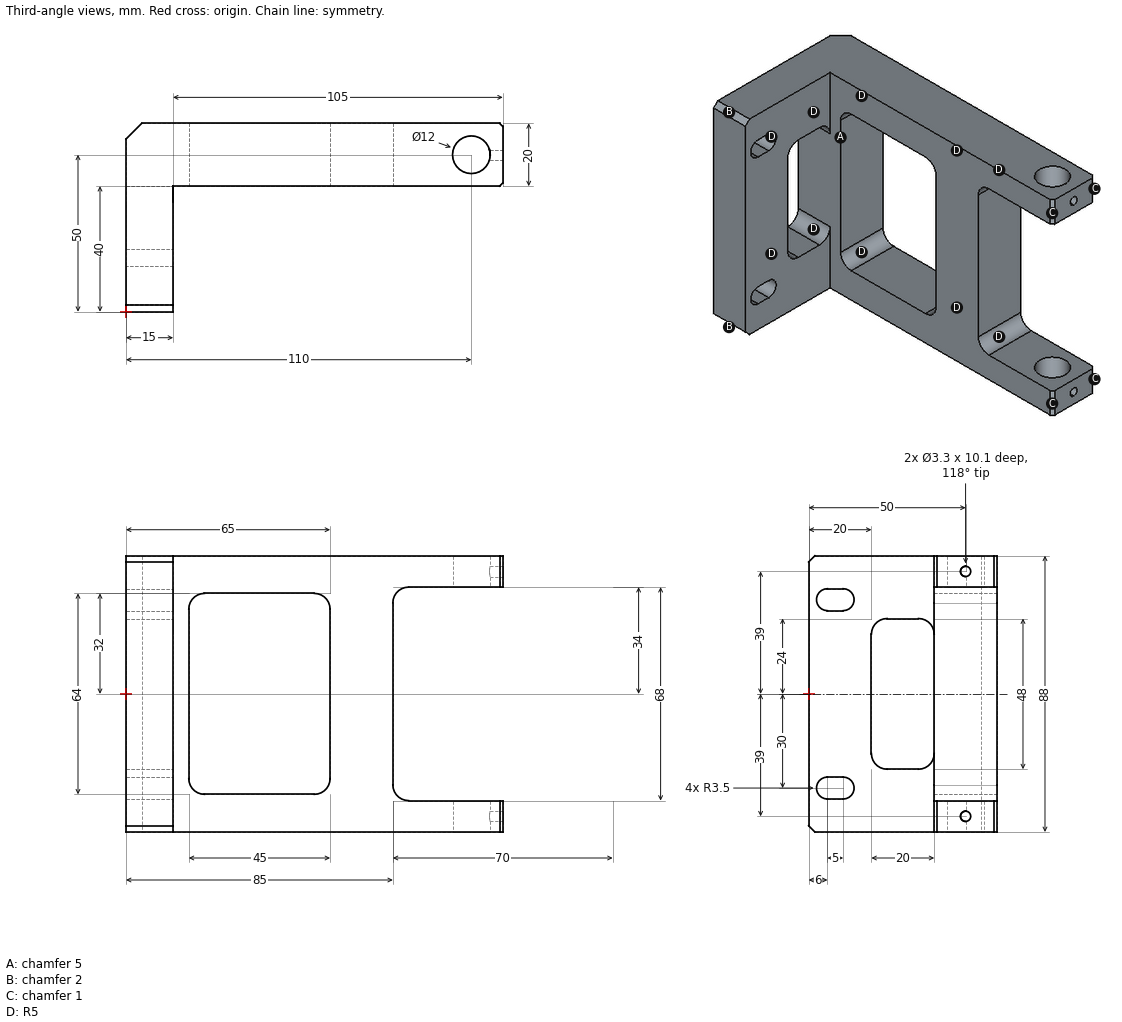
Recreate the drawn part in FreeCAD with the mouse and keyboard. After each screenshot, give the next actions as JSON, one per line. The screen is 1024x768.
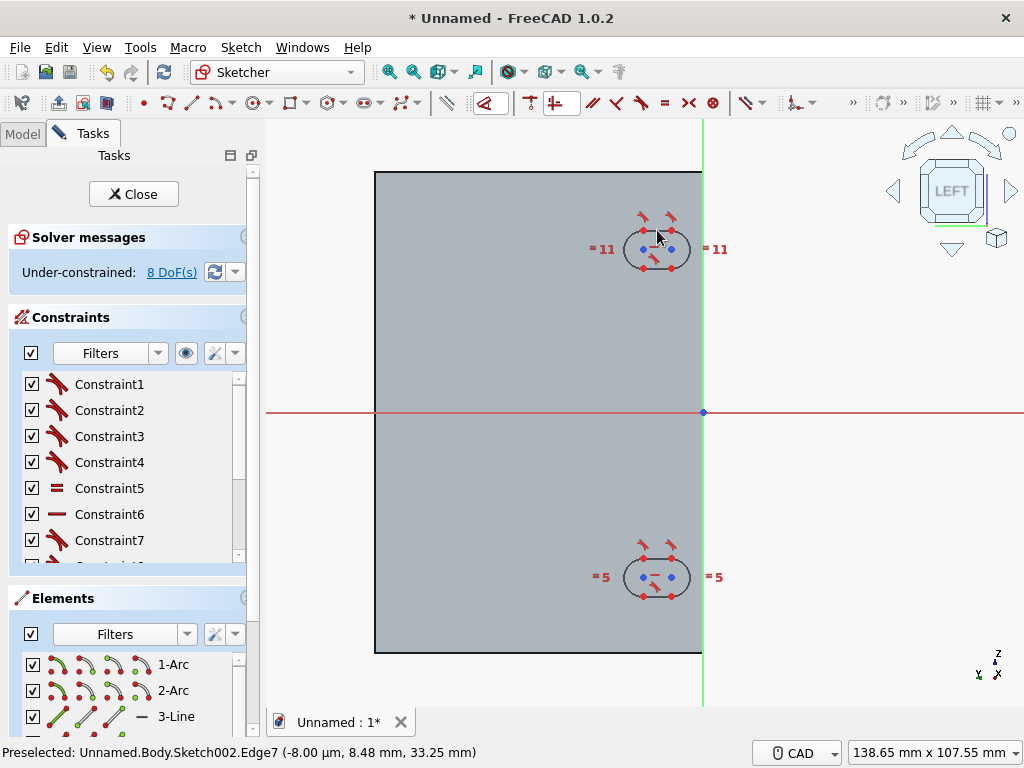
{"action": "left_click", "coordinate": [628, 567]}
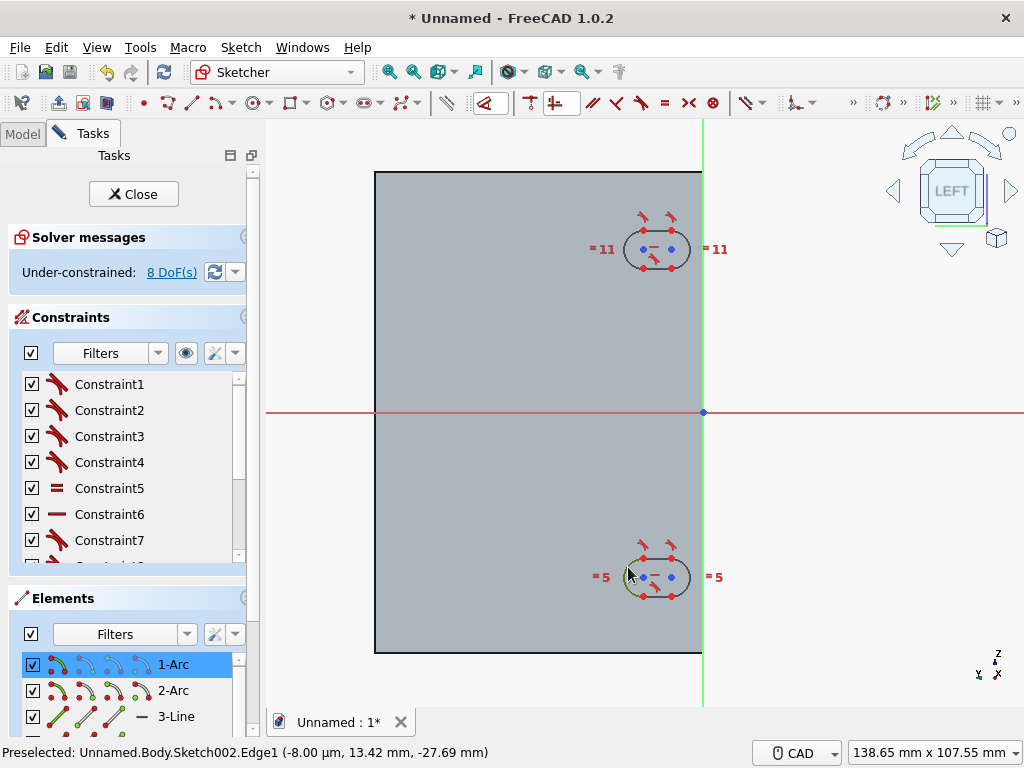
{"action": "left_click", "coordinate": [628, 239]}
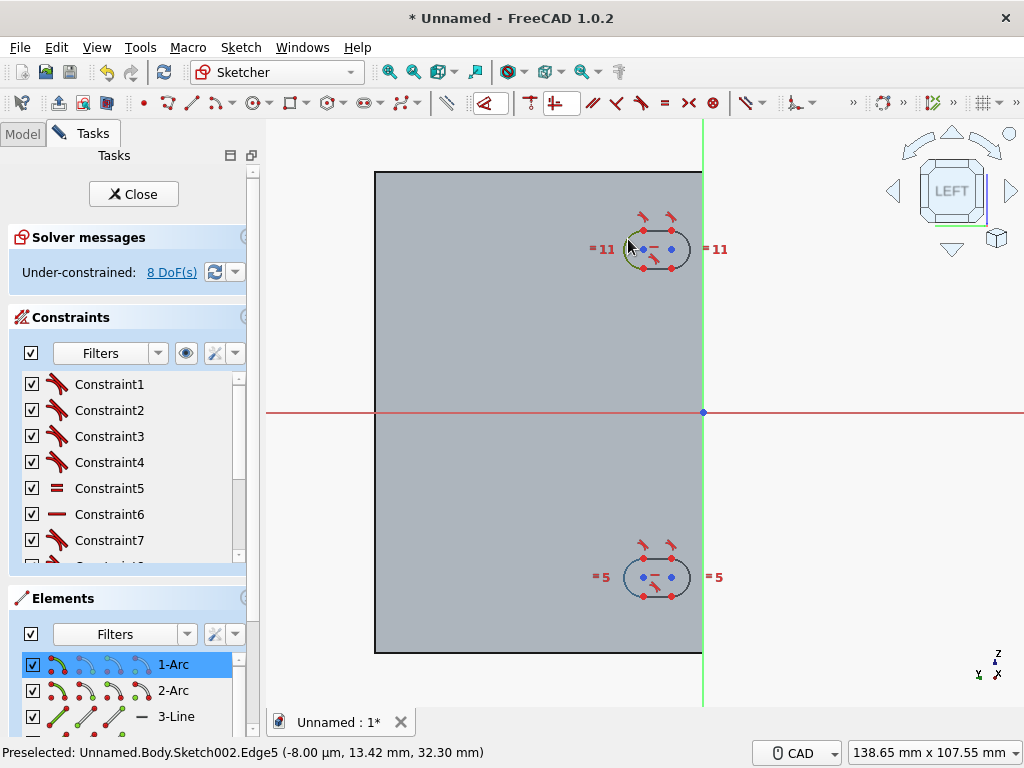
{"action": "key", "text": "e"}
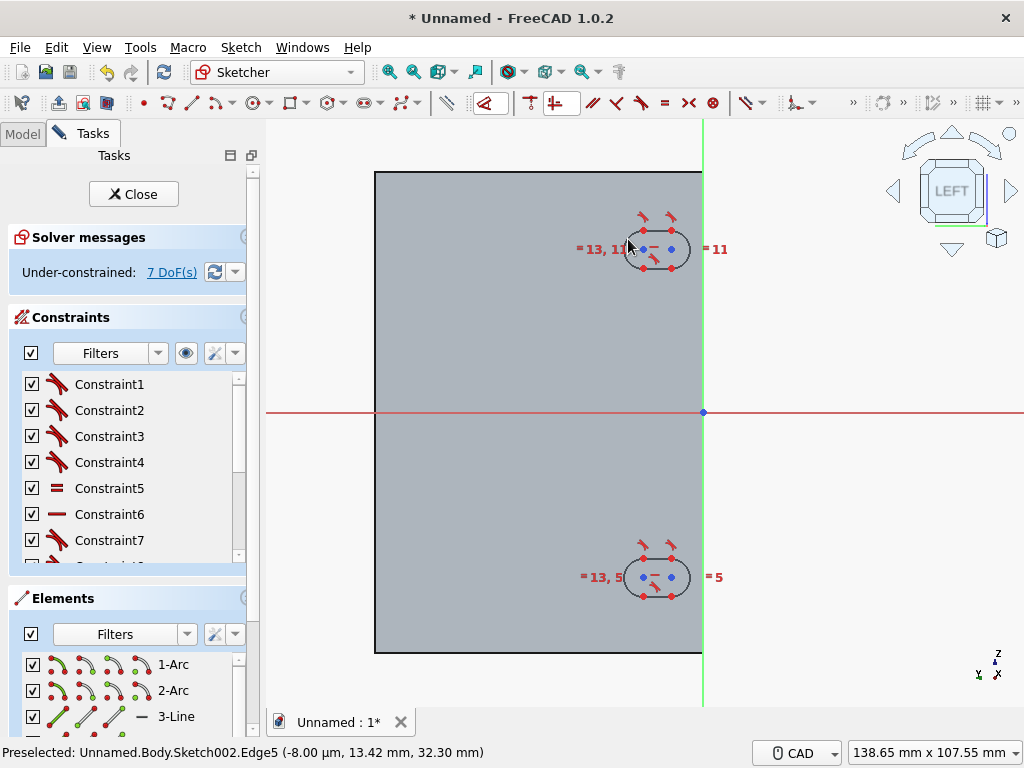
{"action": "left_click", "coordinate": [643, 578]}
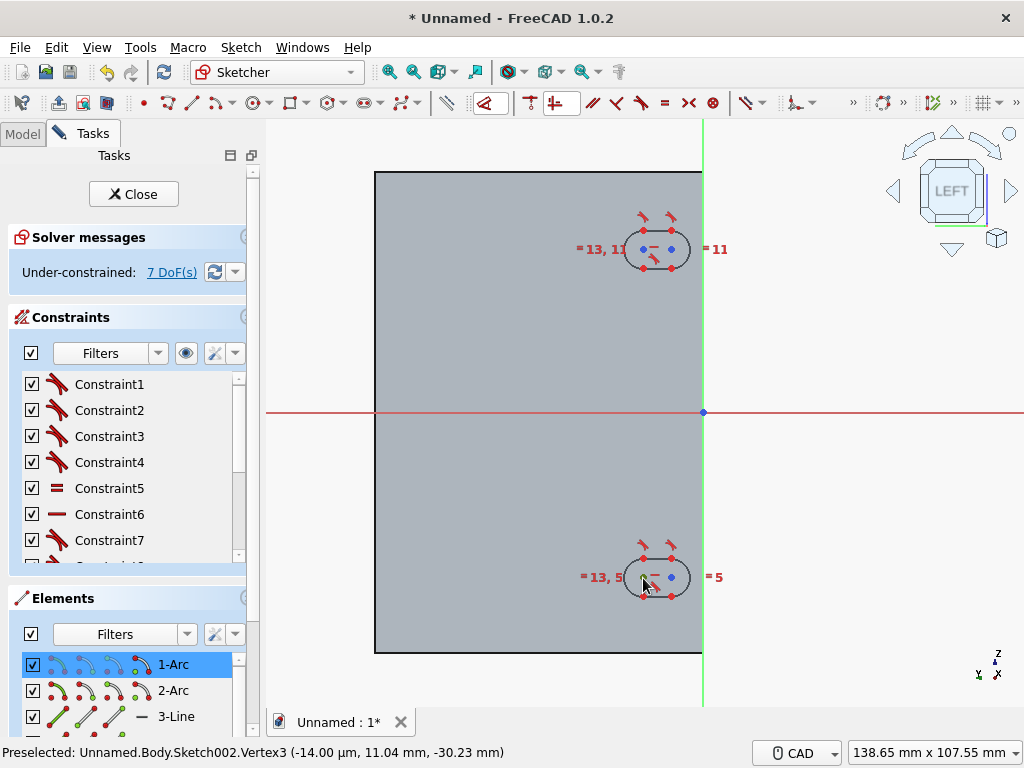
{"action": "left_click", "coordinate": [643, 250]}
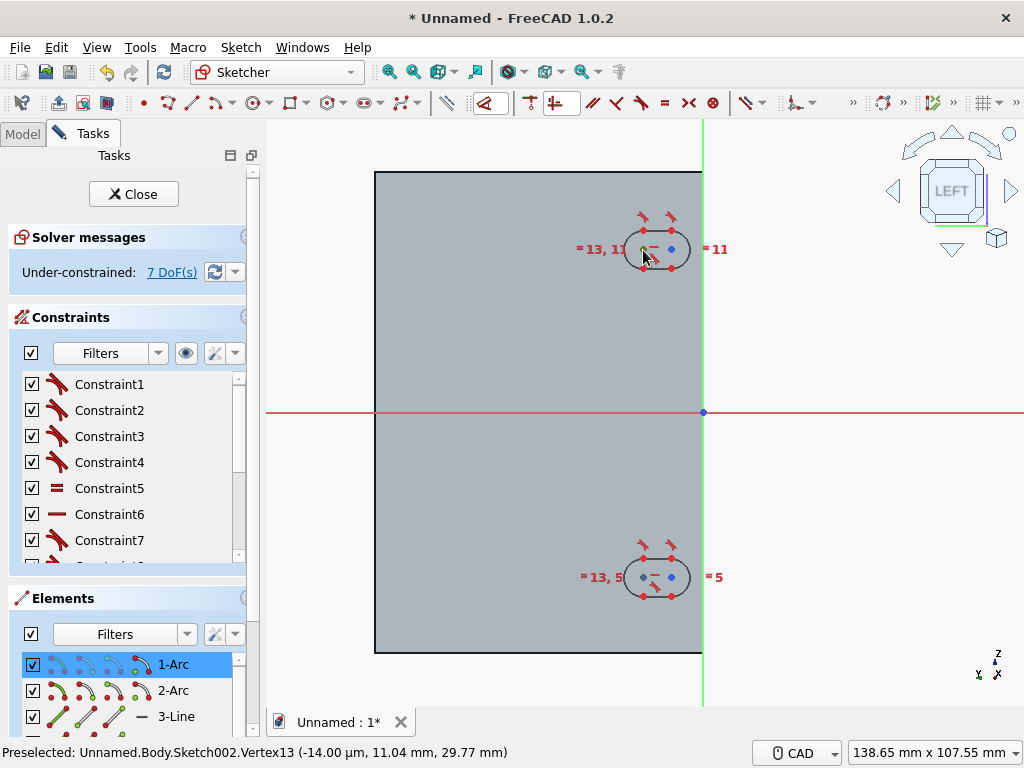
{"action": "left_click", "coordinate": [334, 413]}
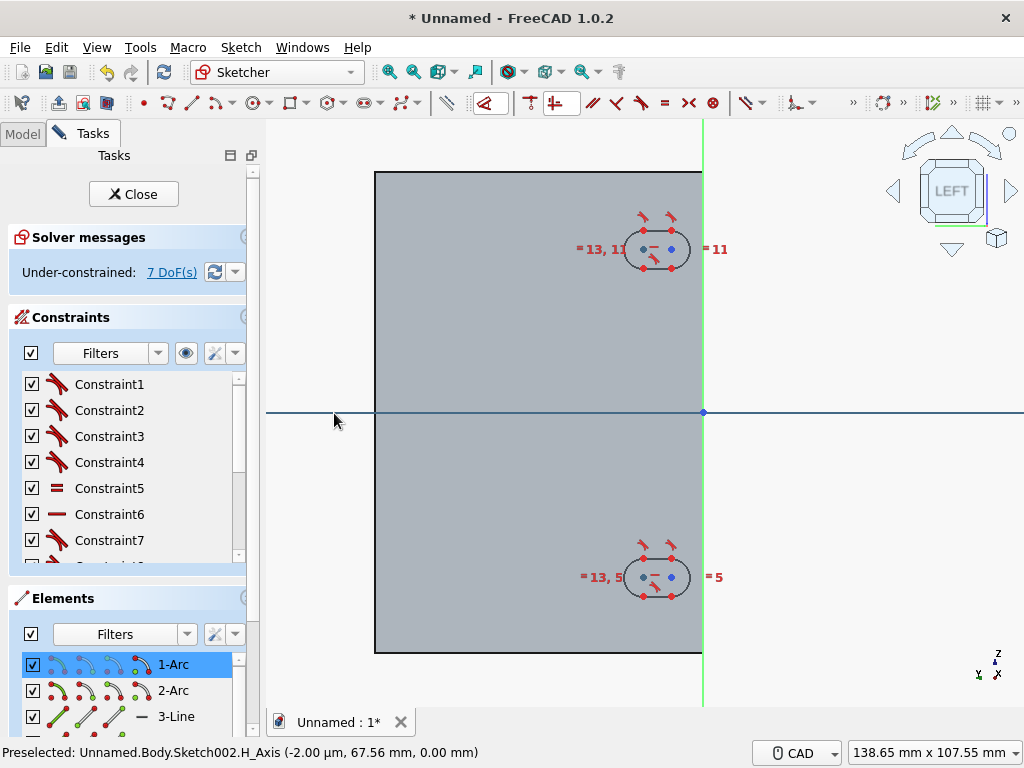
{"action": "key", "text": "s"}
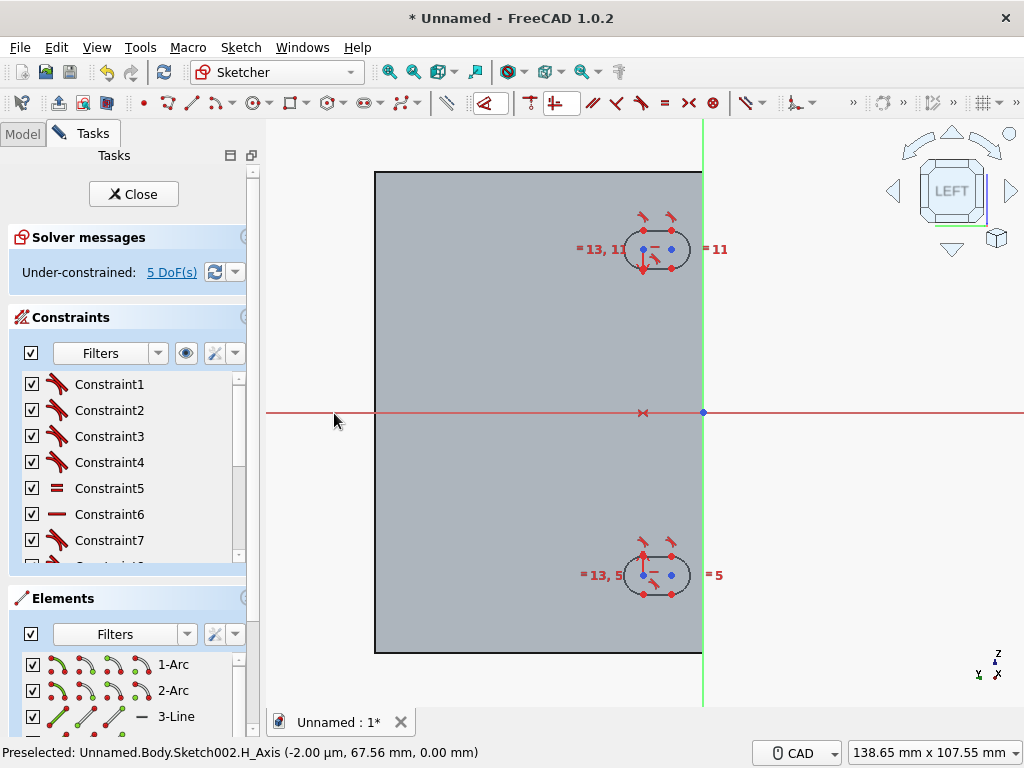
{"action": "scroll", "coordinate": [628, 564], "scroll_direction": "up", "scroll_amount": 4}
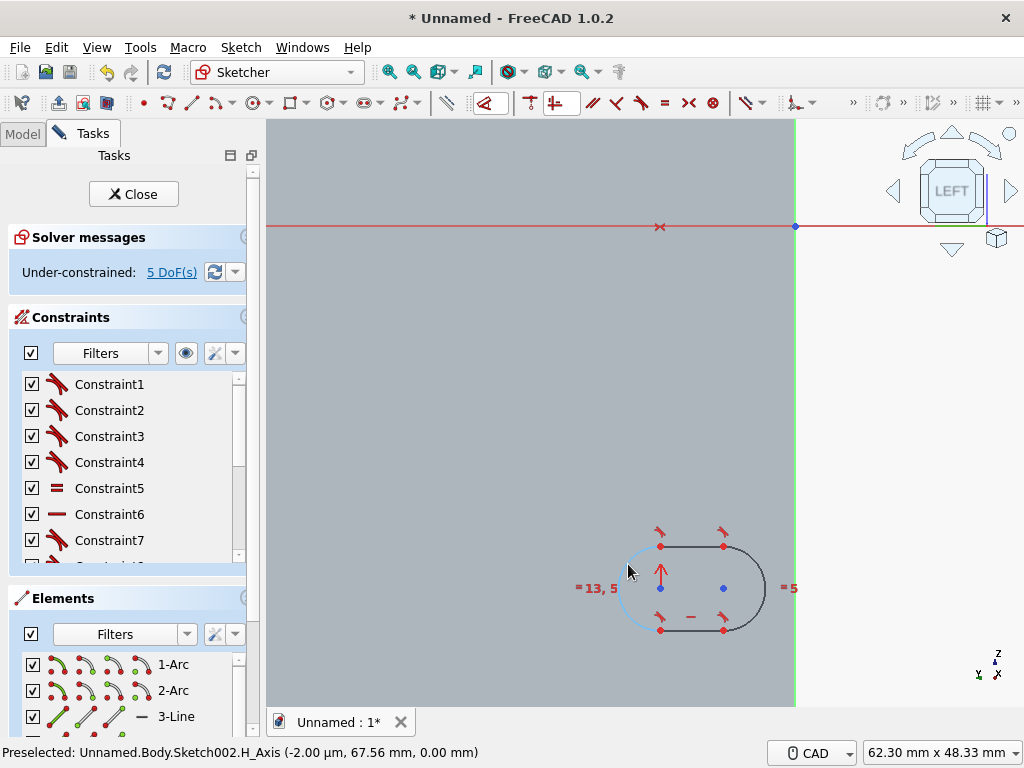
{"action": "left_click", "coordinate": [627, 564]}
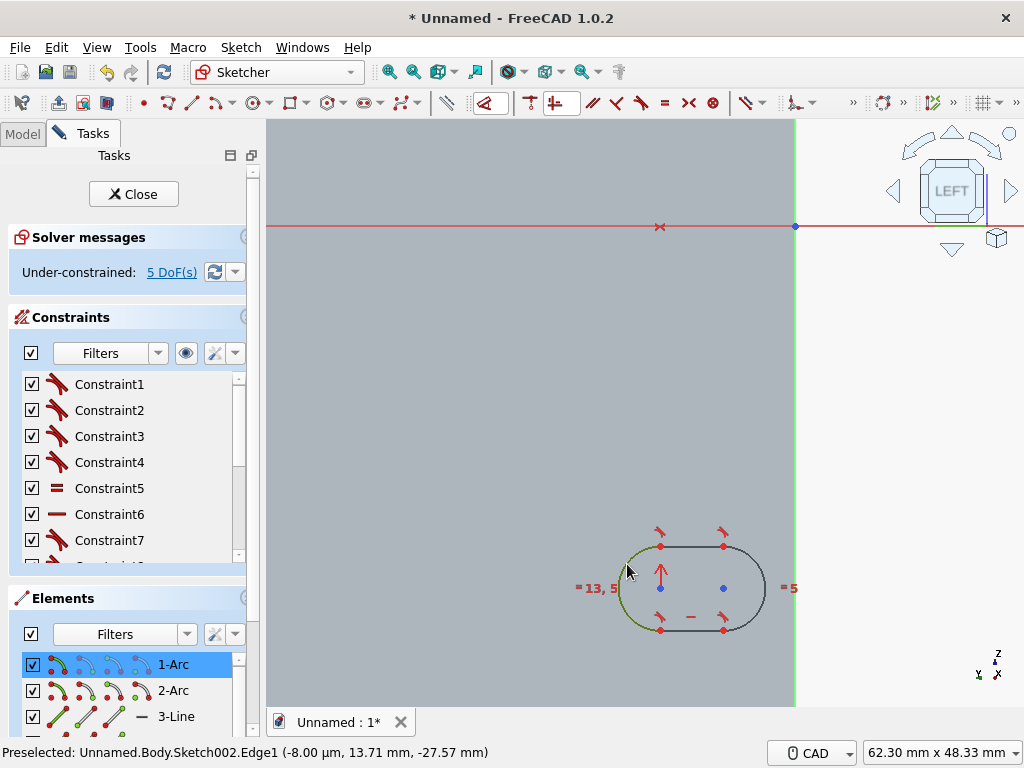
{"action": "key", "text": "k r"}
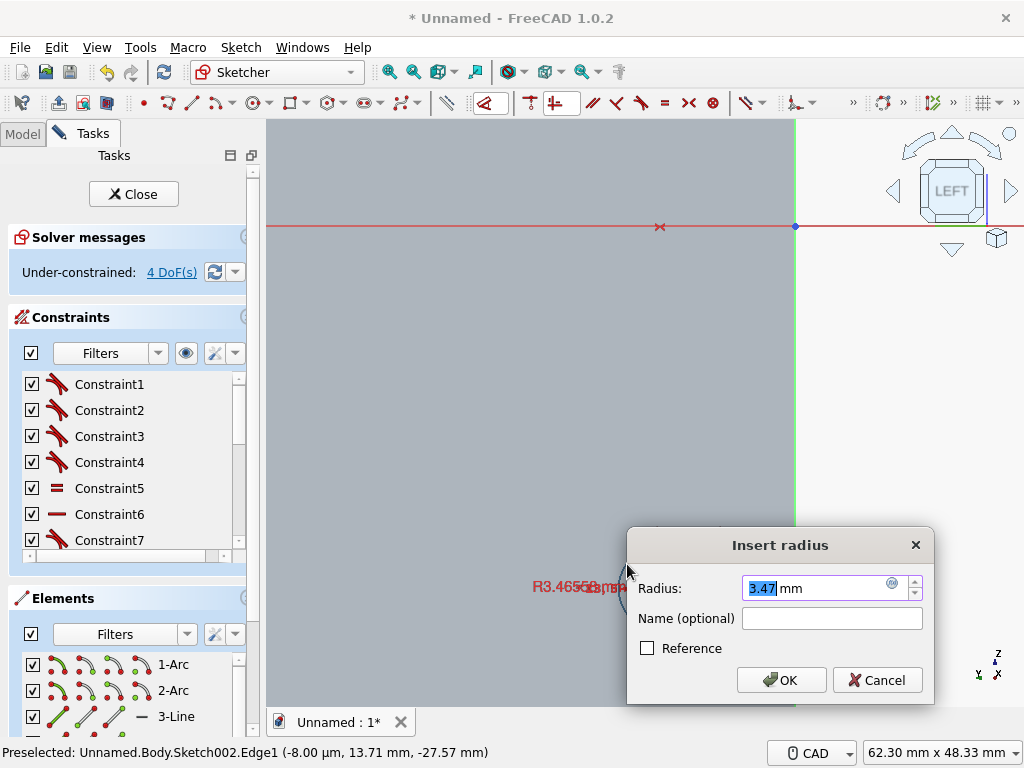
{"action": "type", "text": "3.5"}
{"action": "key", "text": "Return"}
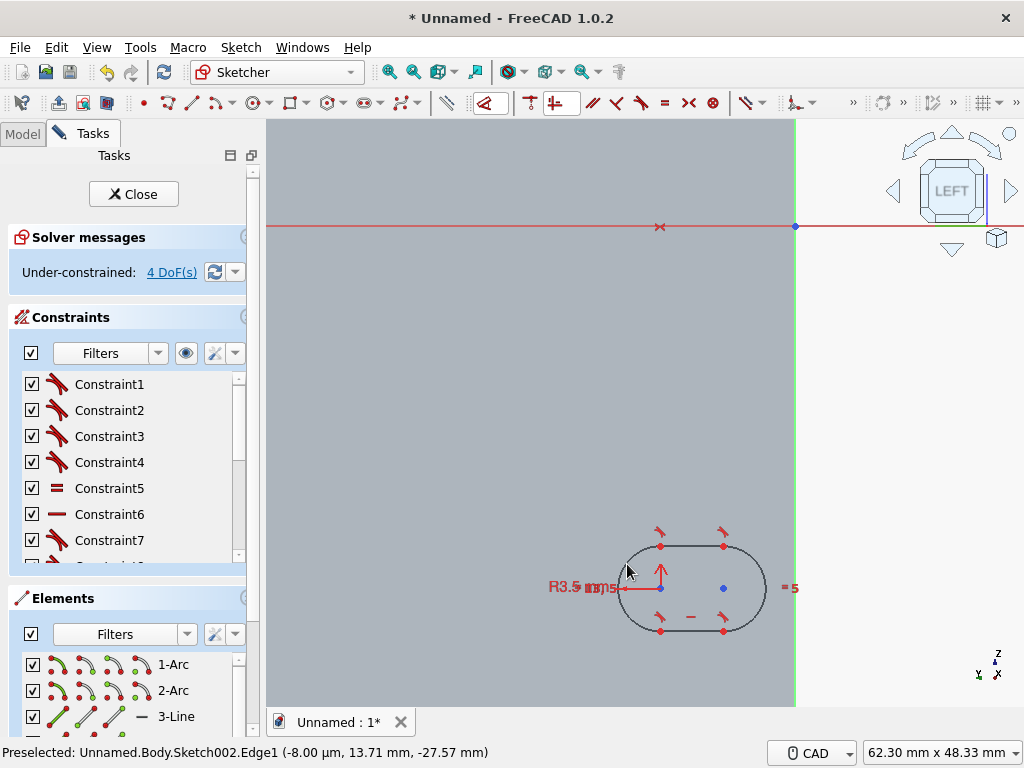
{"action": "left_click", "coordinate": [679, 546]}